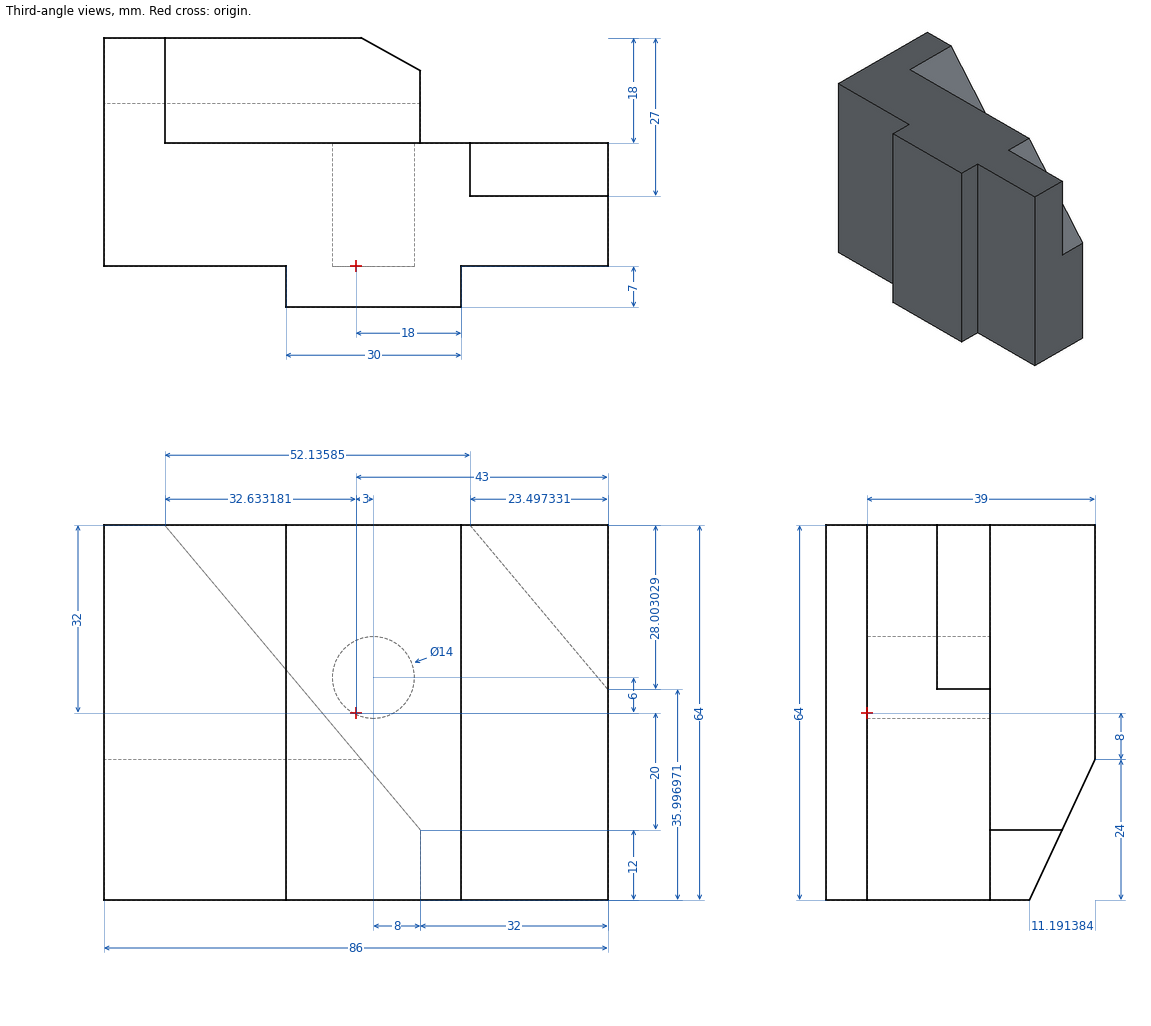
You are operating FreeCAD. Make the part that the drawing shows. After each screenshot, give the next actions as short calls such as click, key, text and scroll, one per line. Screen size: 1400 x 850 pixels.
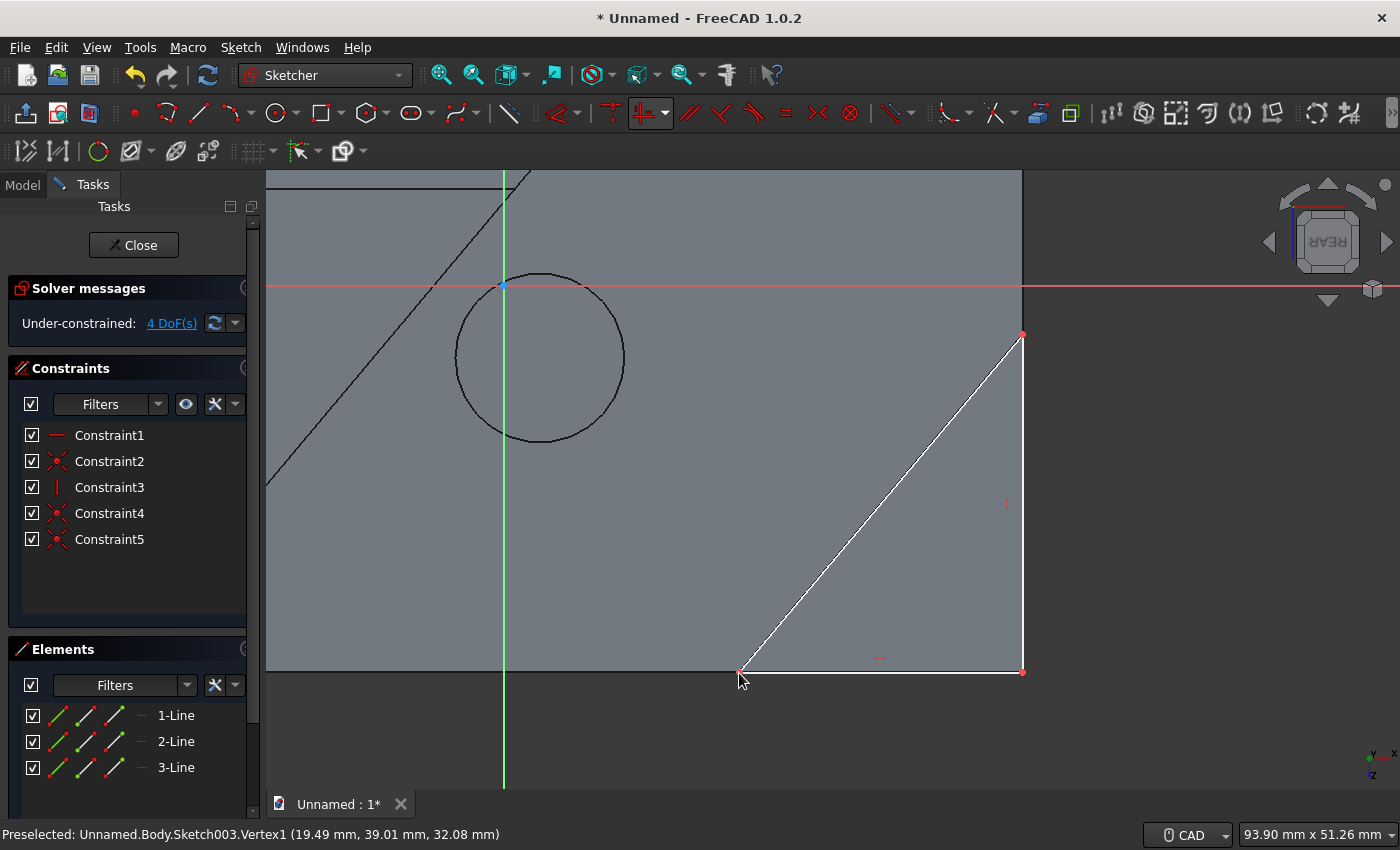
key(d)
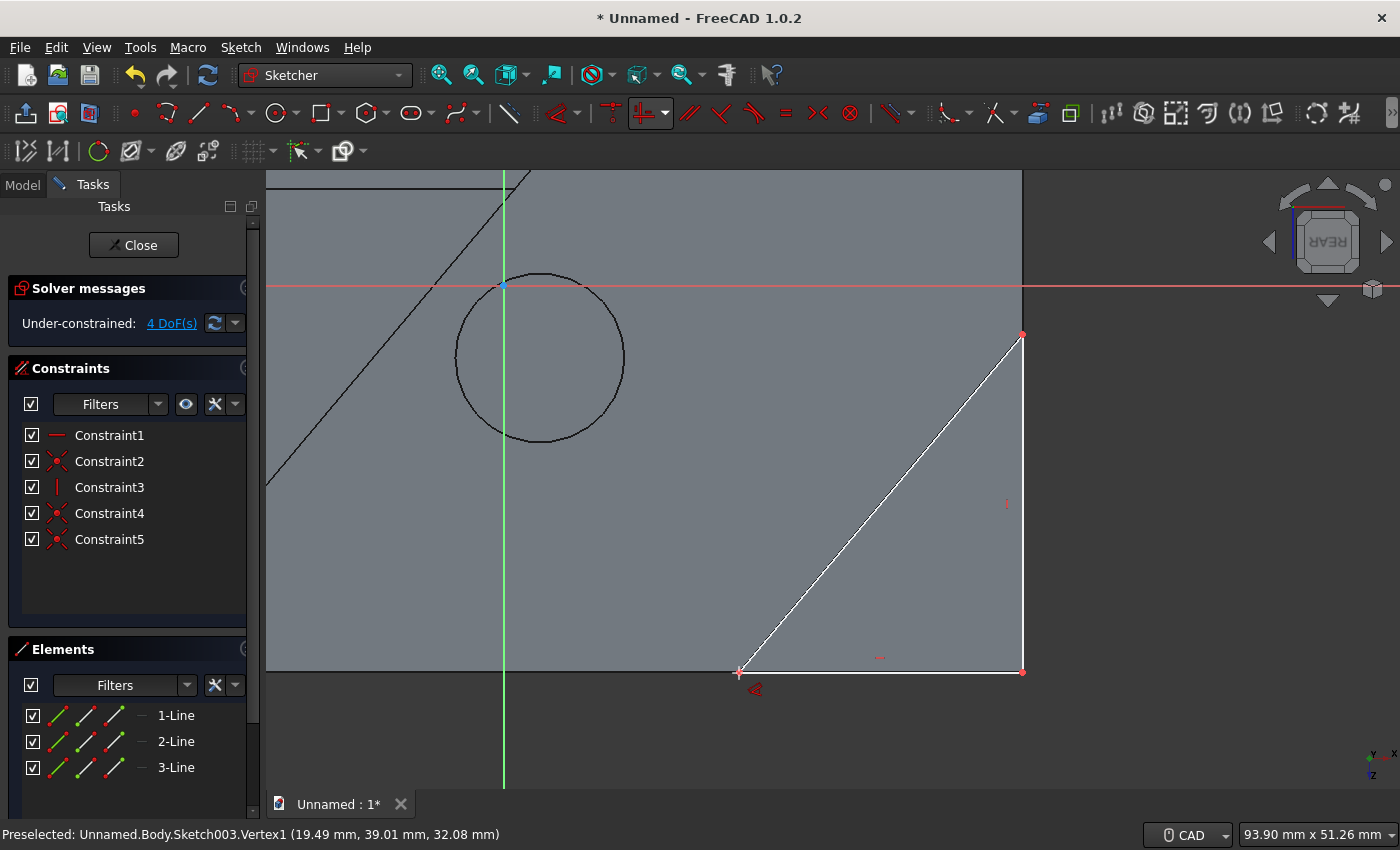
click(739, 673)
click(470, 479)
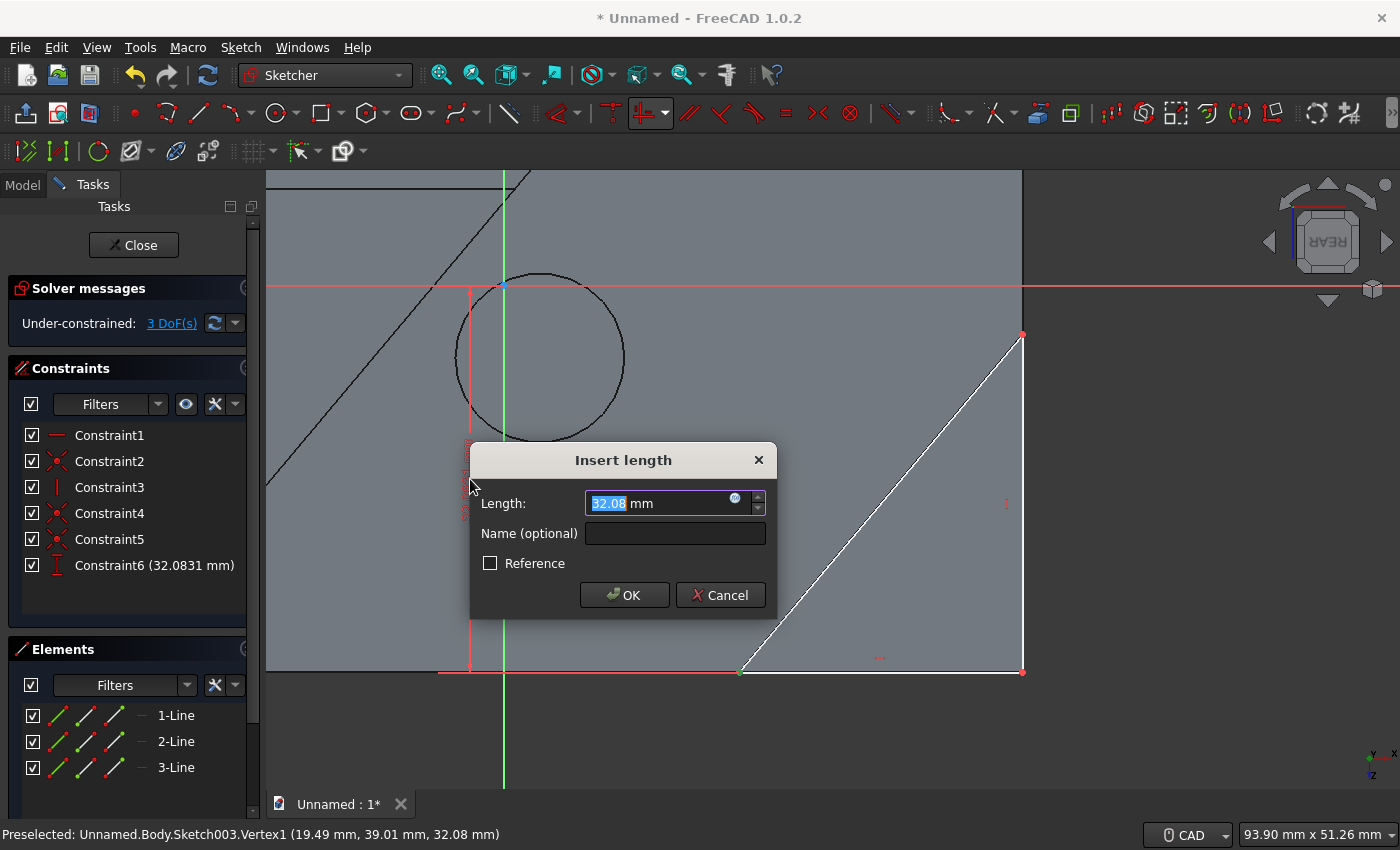
text(32)
key(Return)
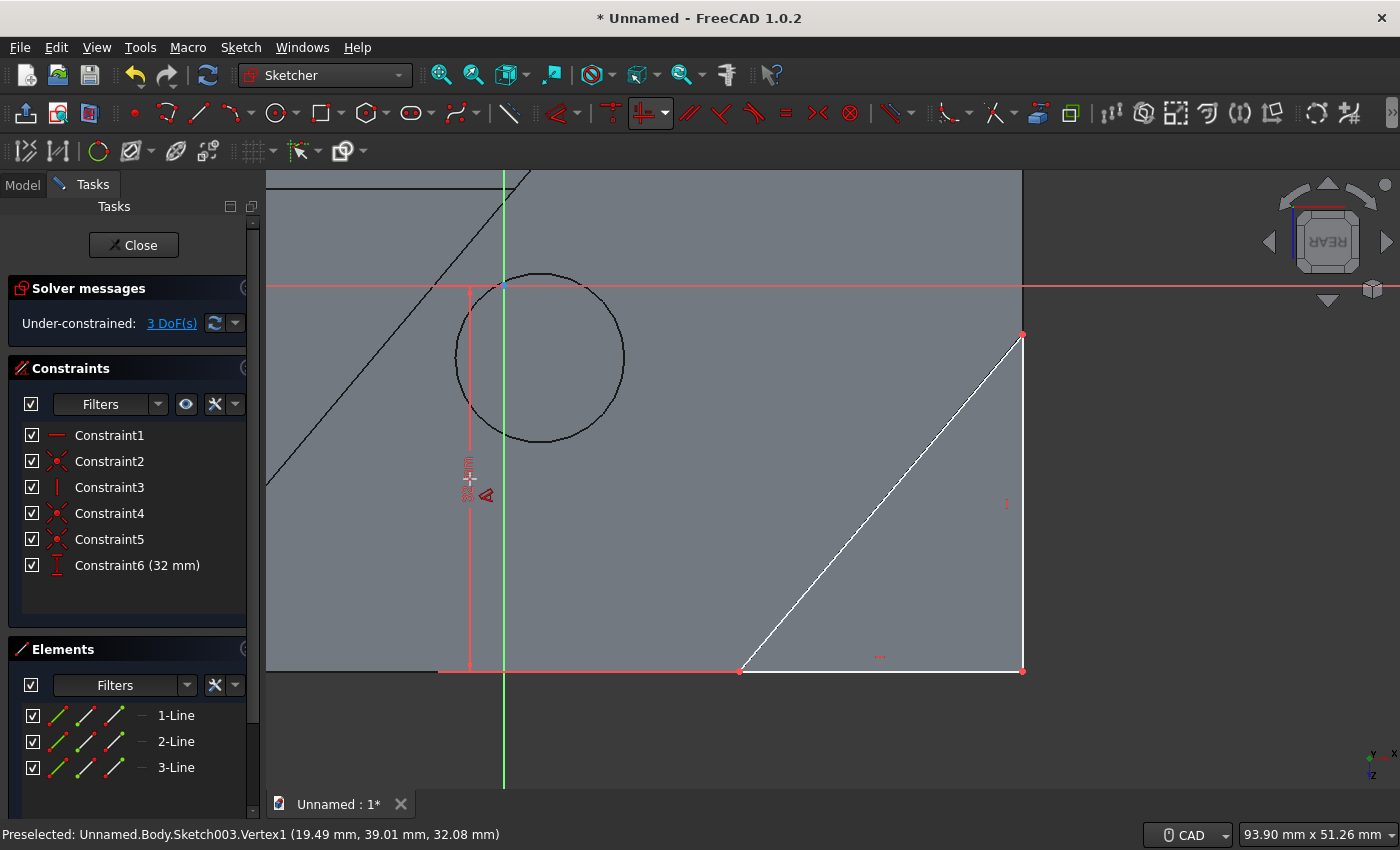
click(1023, 672)
click(763, 706)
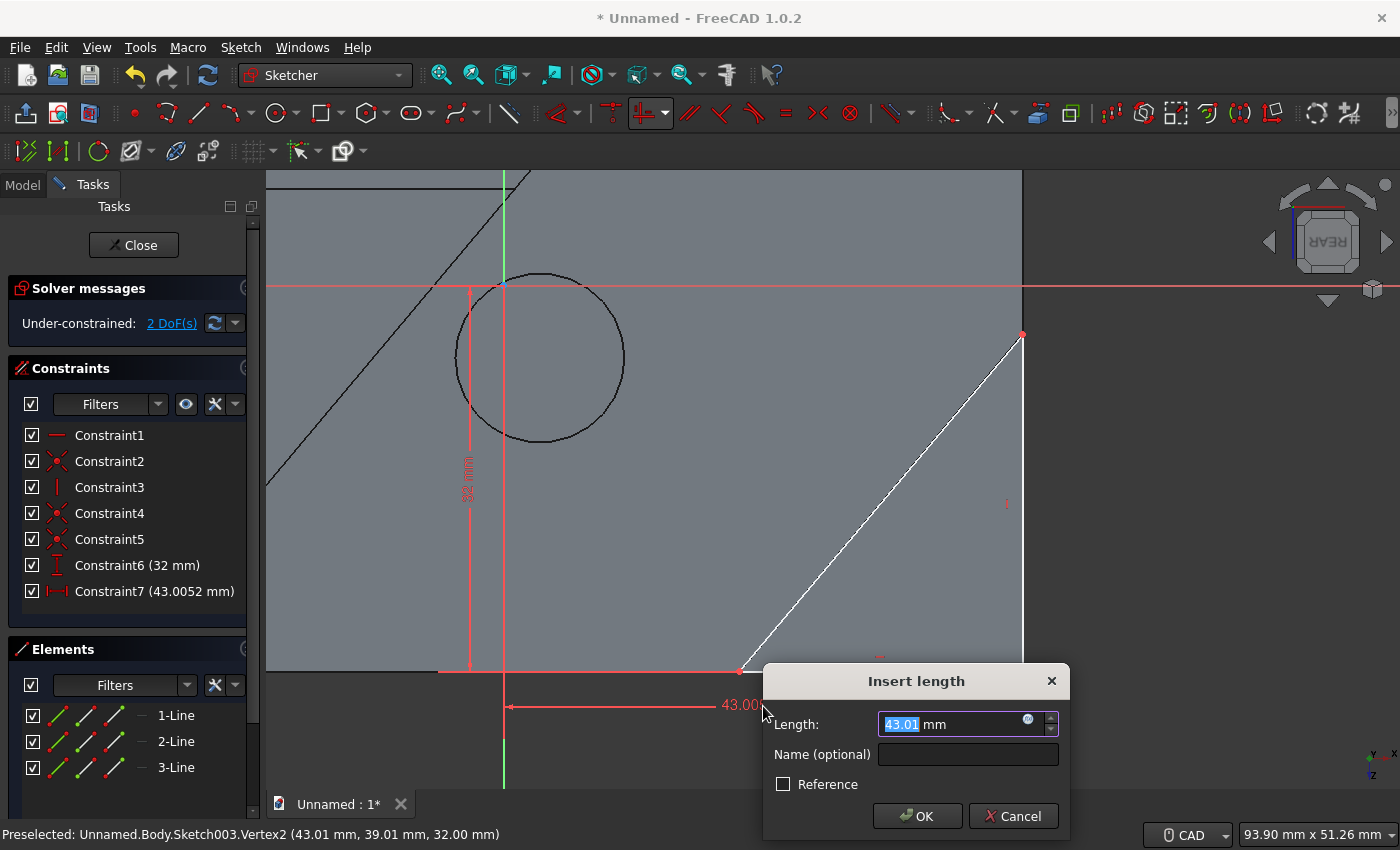
text(43)
key(Return)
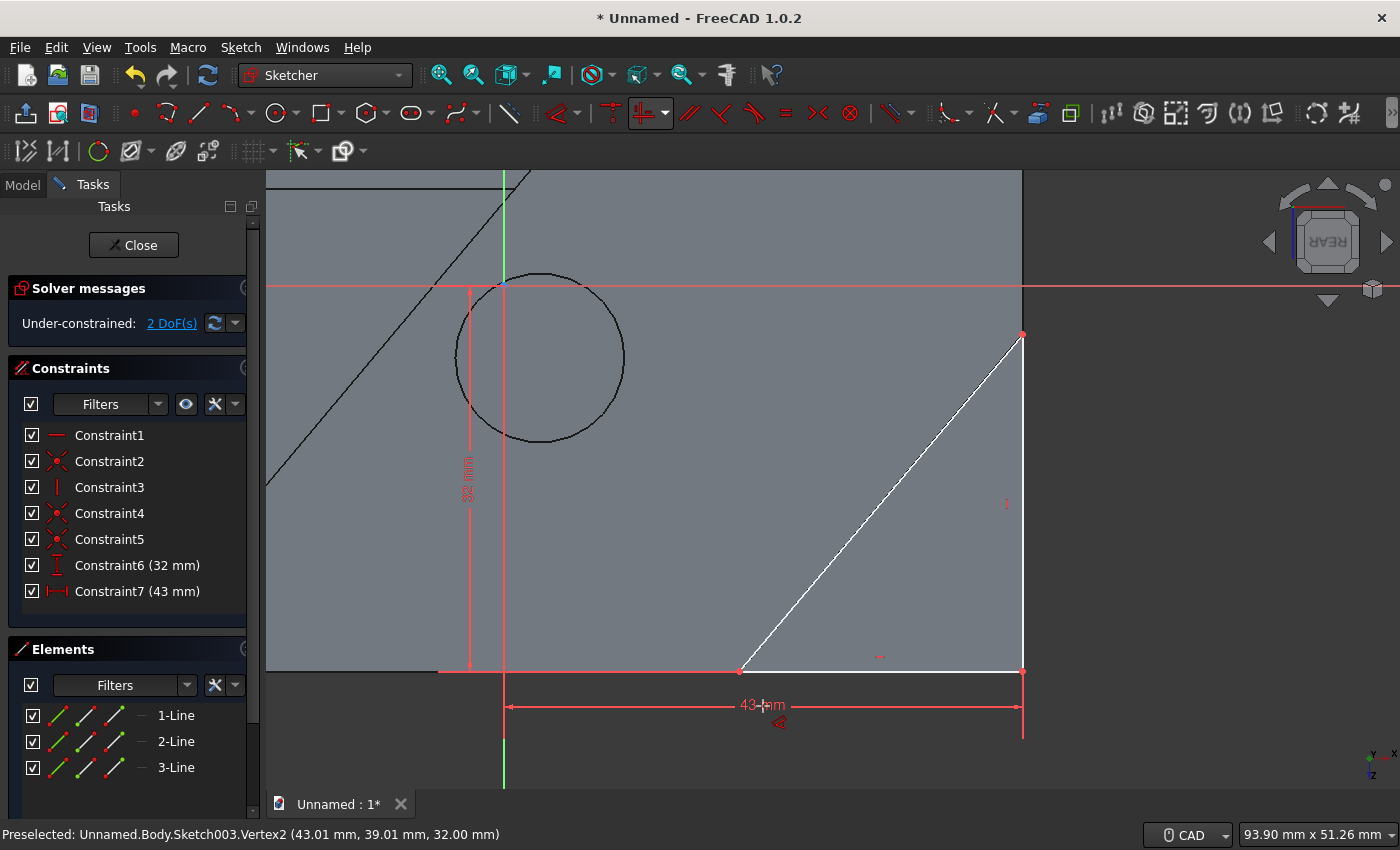
click(824, 672)
click(881, 706)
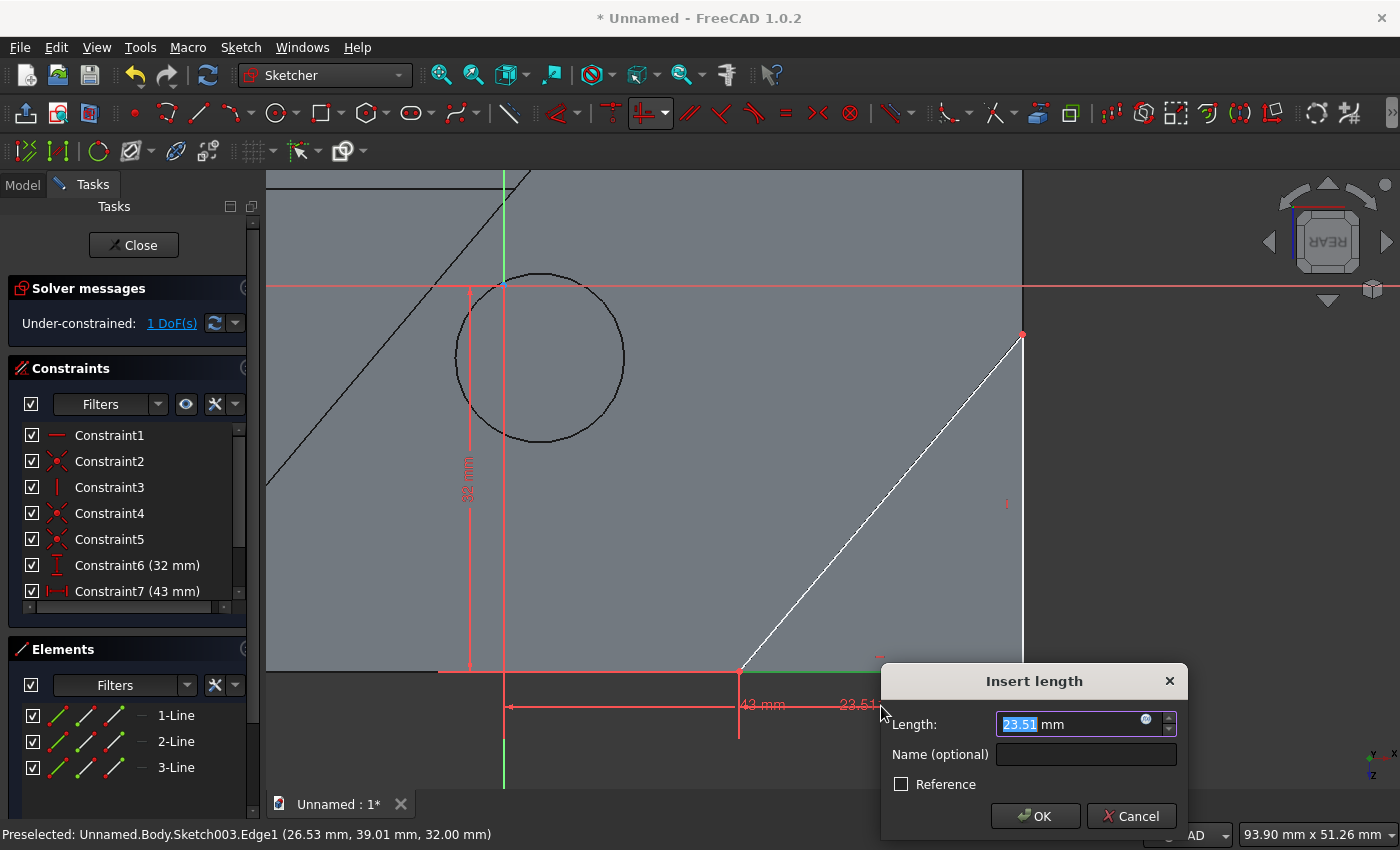
text(23.497331)
key(Return)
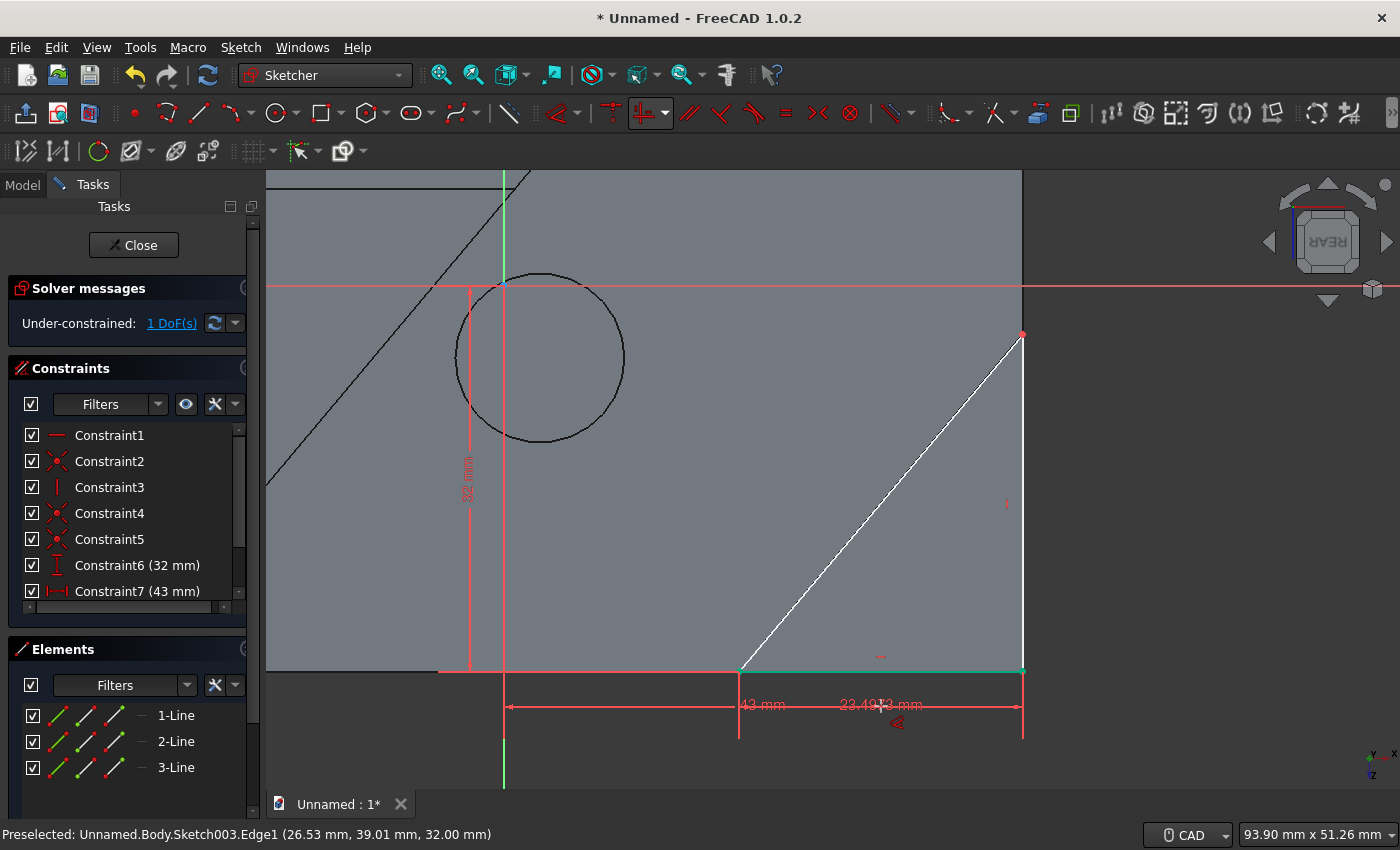
click(1023, 571)
click(1057, 503)